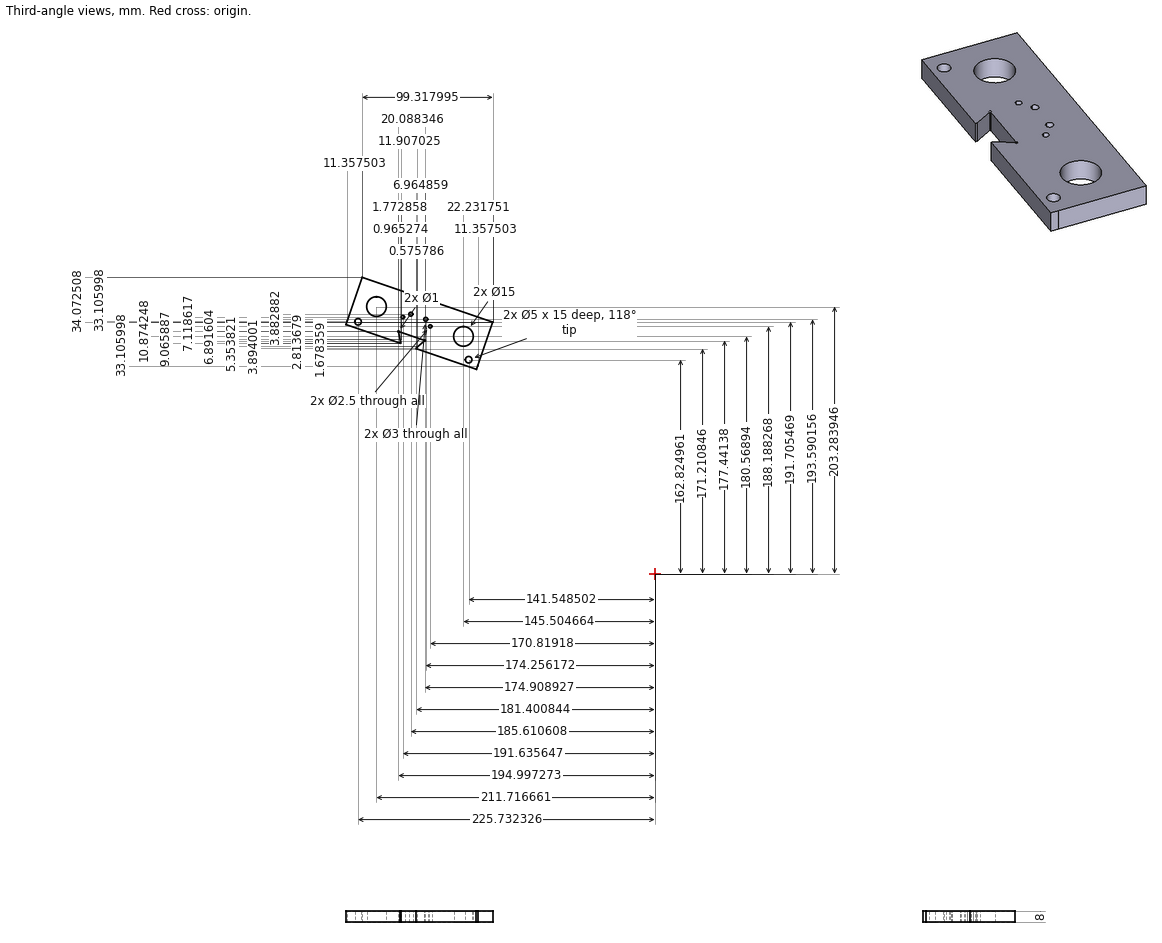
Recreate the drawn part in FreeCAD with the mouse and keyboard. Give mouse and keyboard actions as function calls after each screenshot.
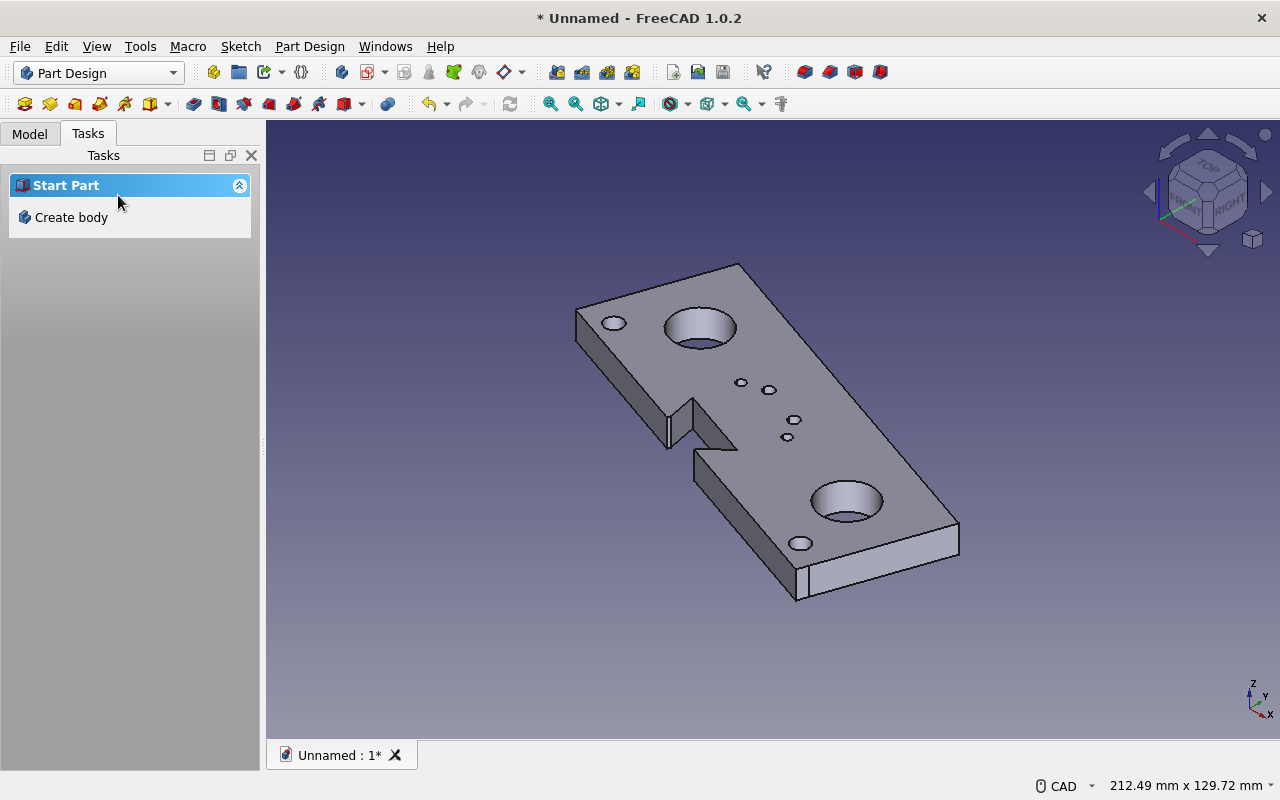
click(787, 466)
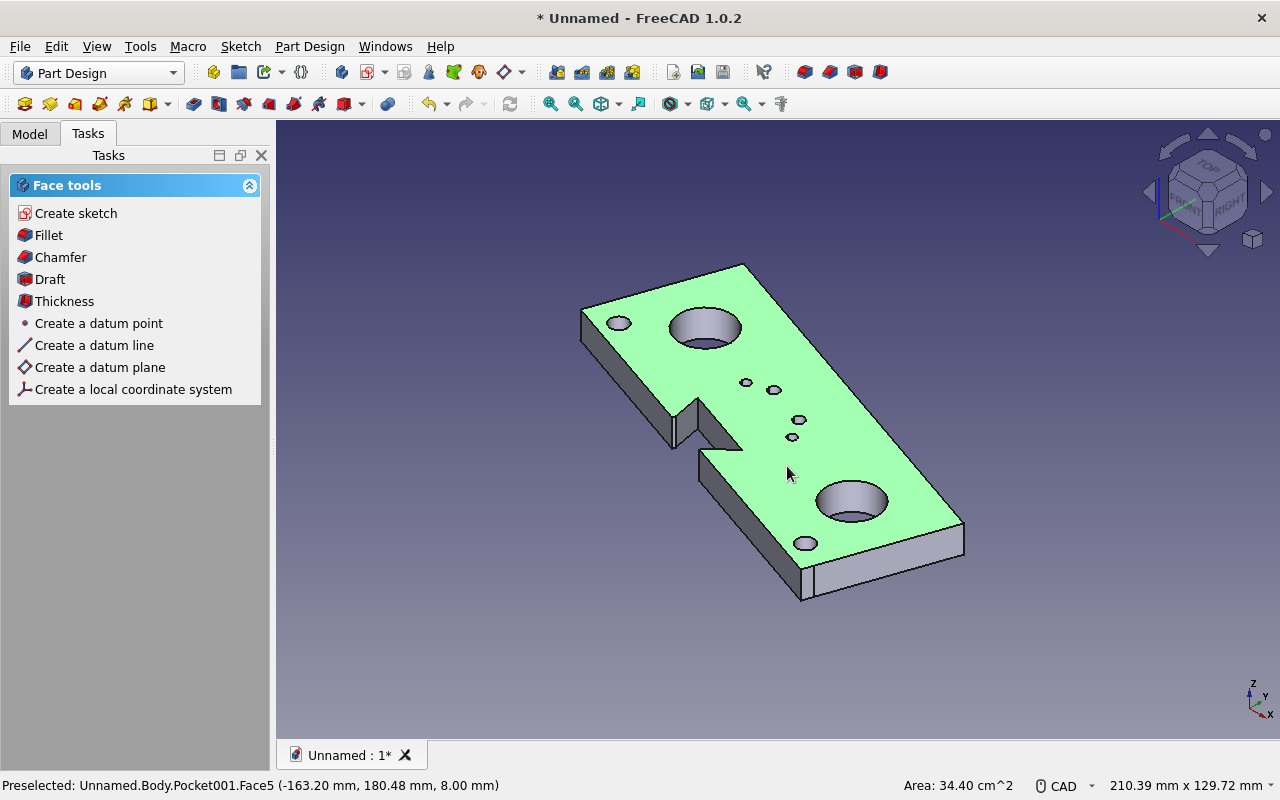
click(366, 72)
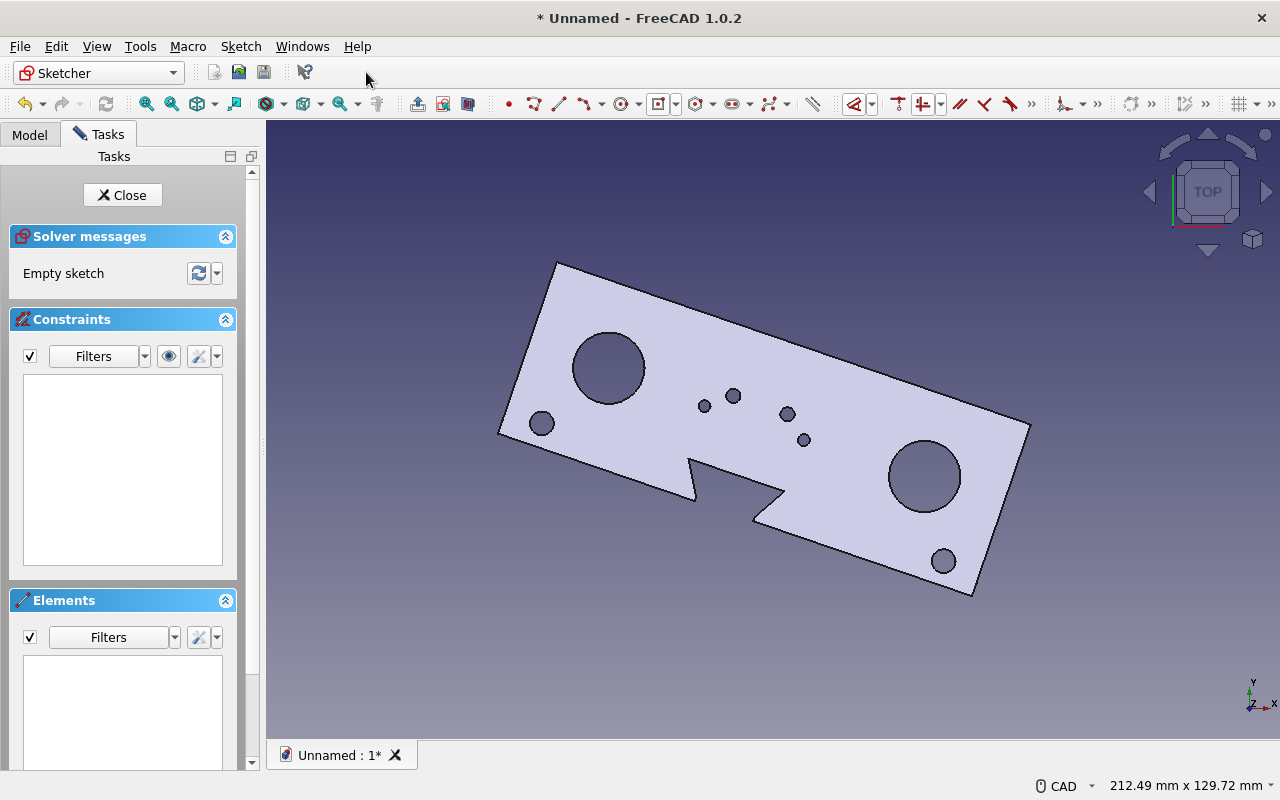
scroll(743, 484, up, 9)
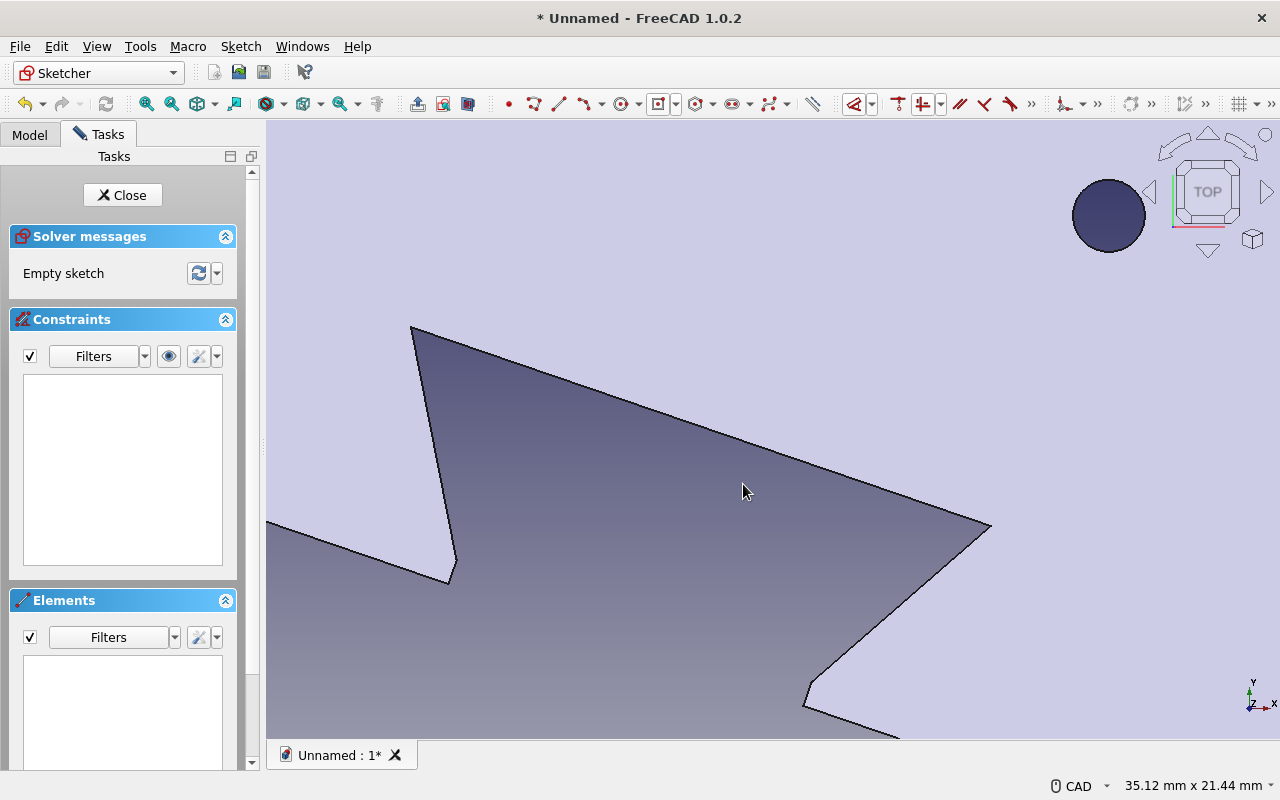
click(620, 104)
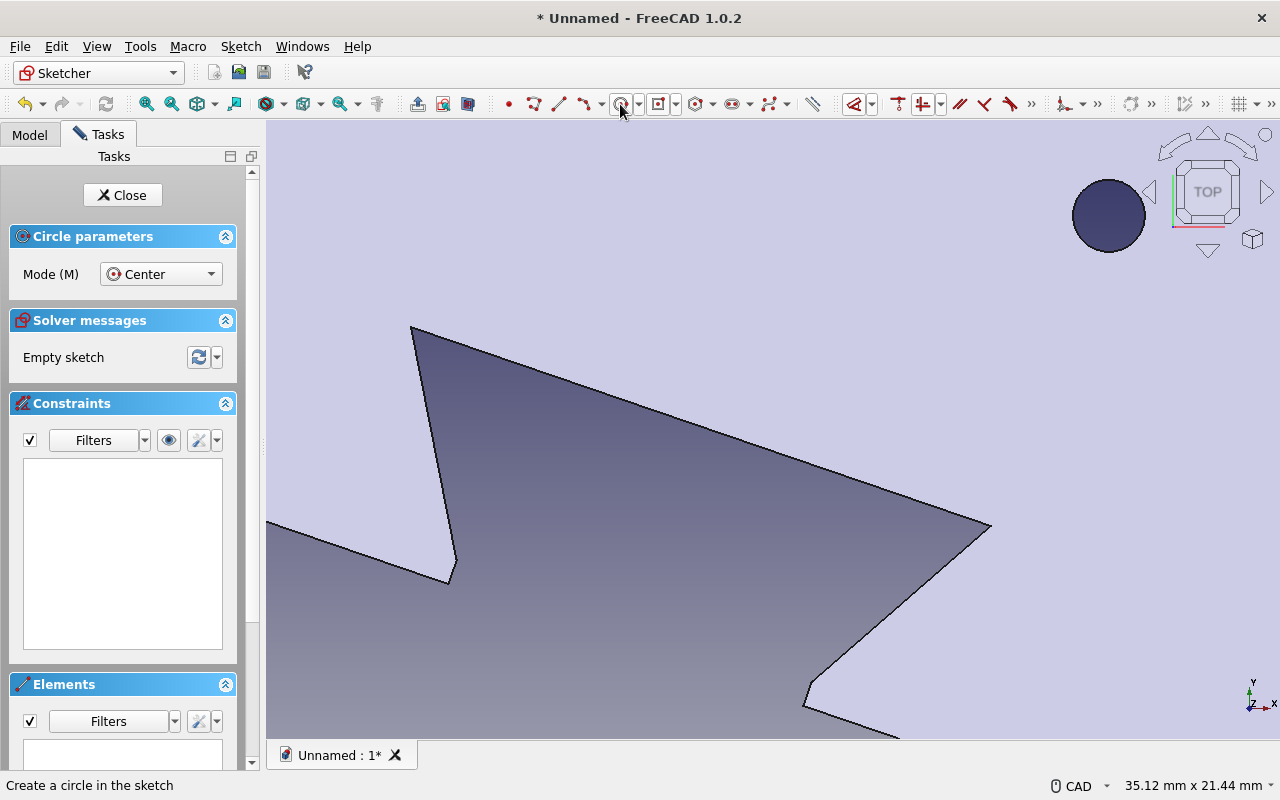
scroll(411, 327, up, 3)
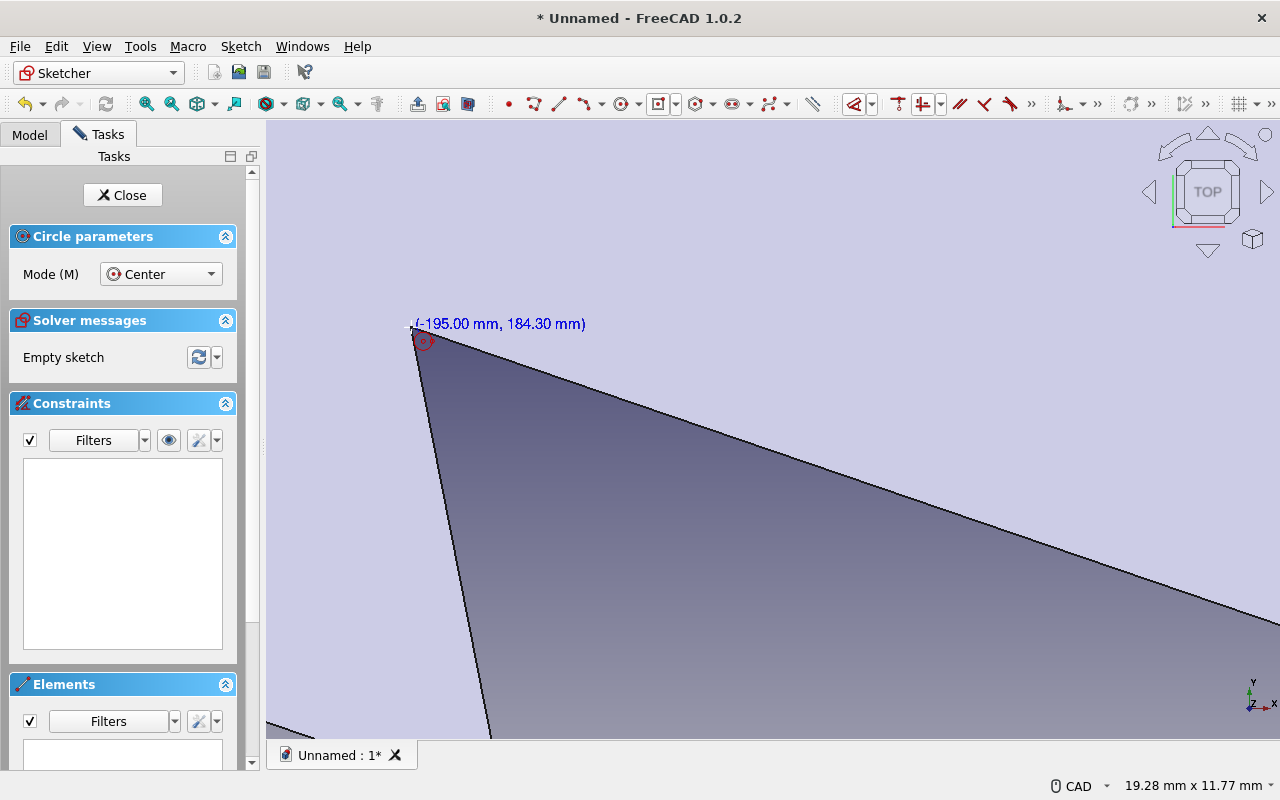
click(411, 327)
click(429, 308)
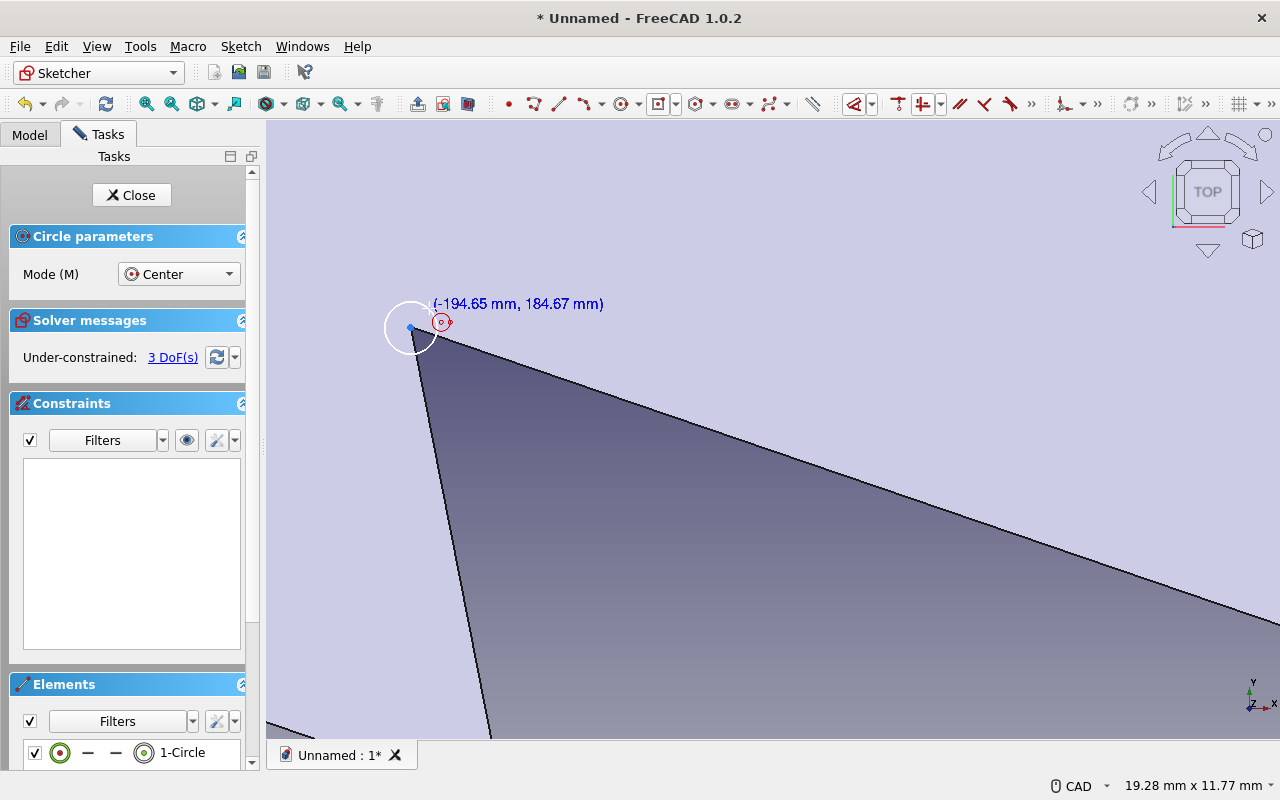
scroll(419, 334, down, 3)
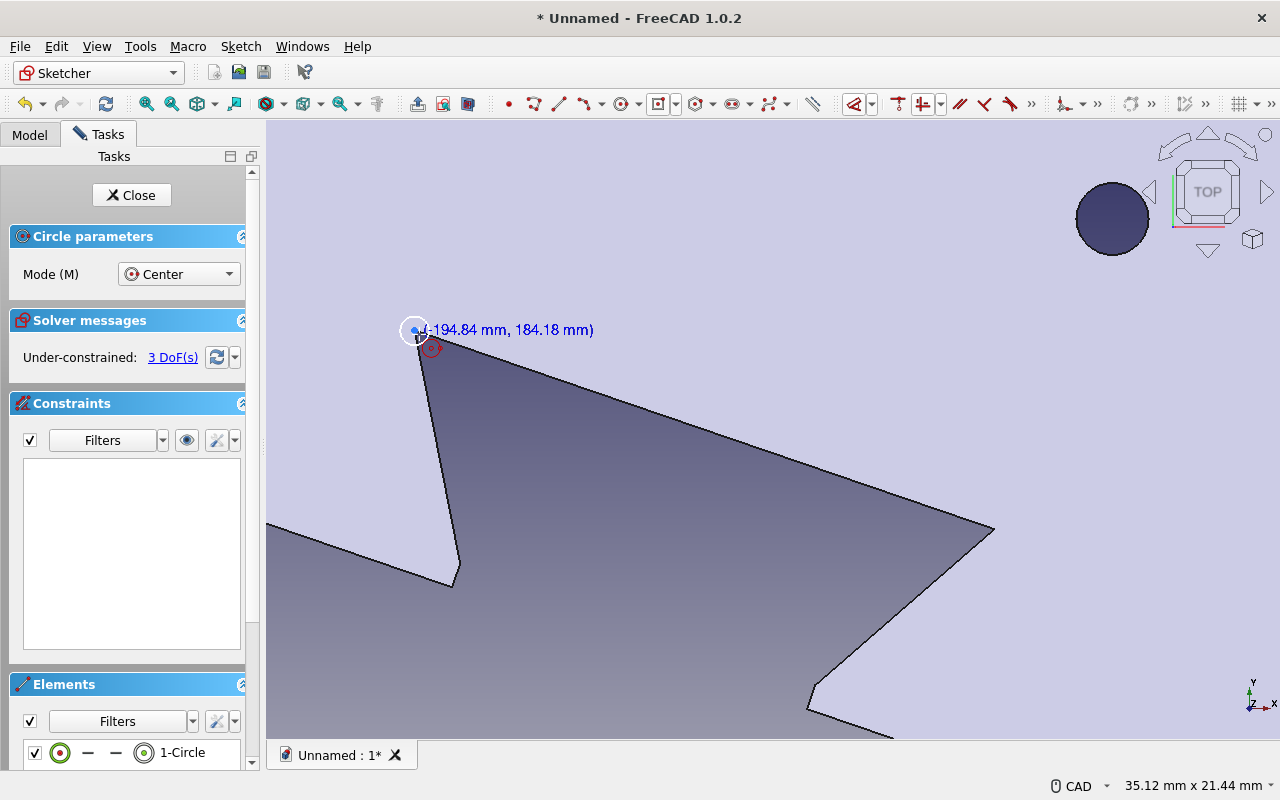
scroll(994, 529, up, 3)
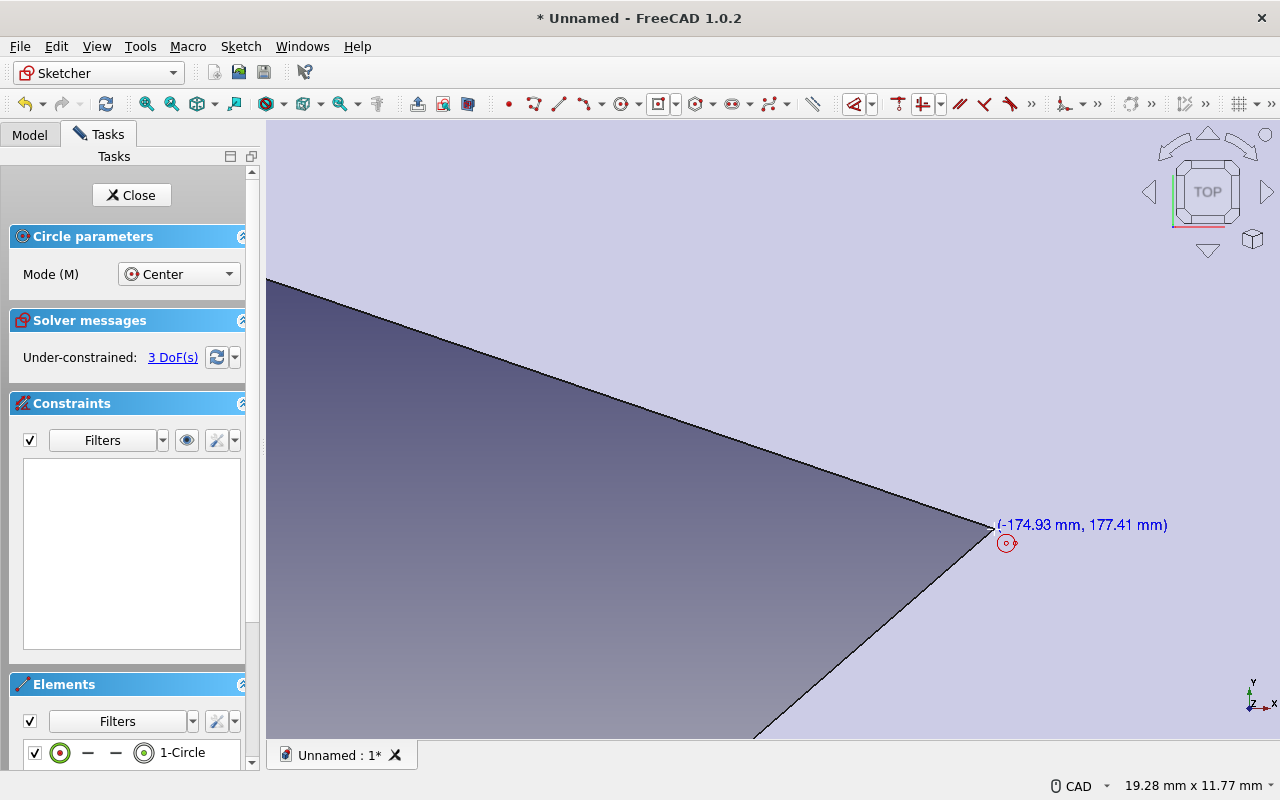
click(994, 529)
click(1013, 510)
key(Escape)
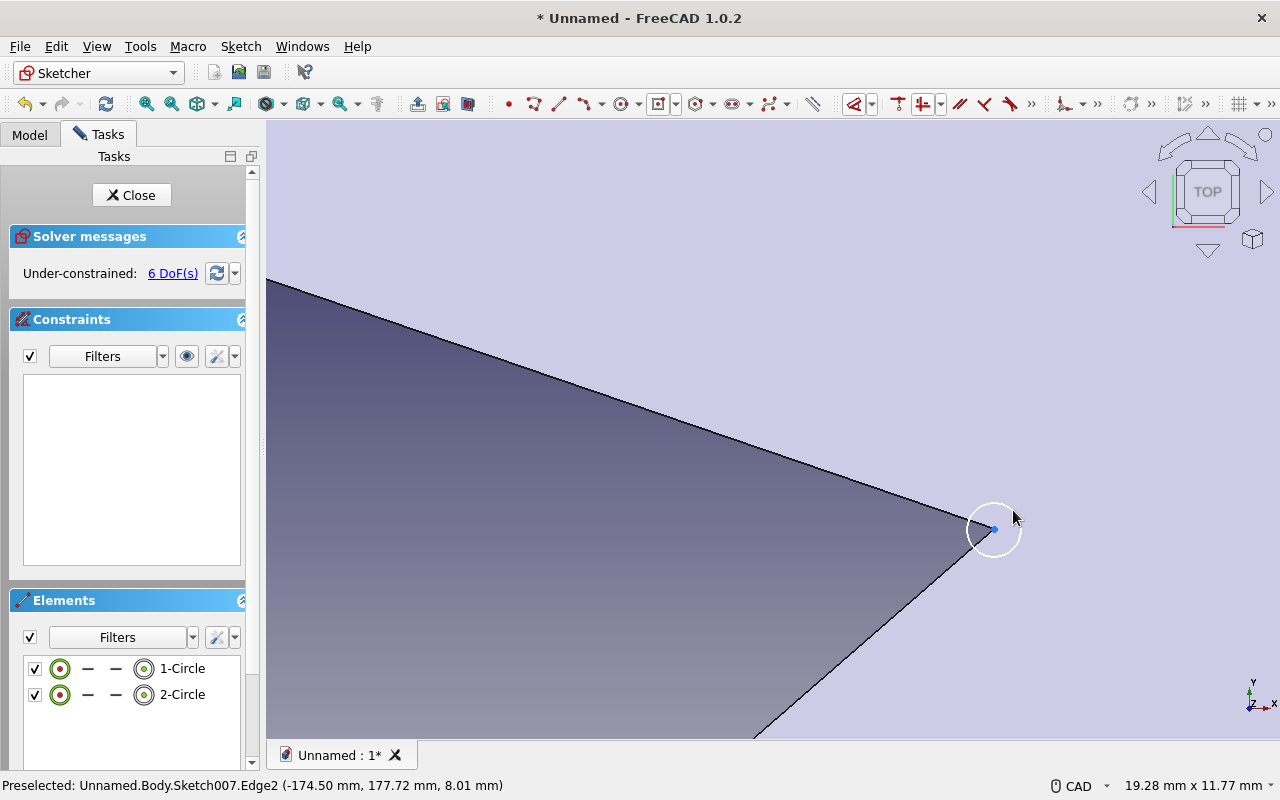
scroll(995, 529, down, 3)